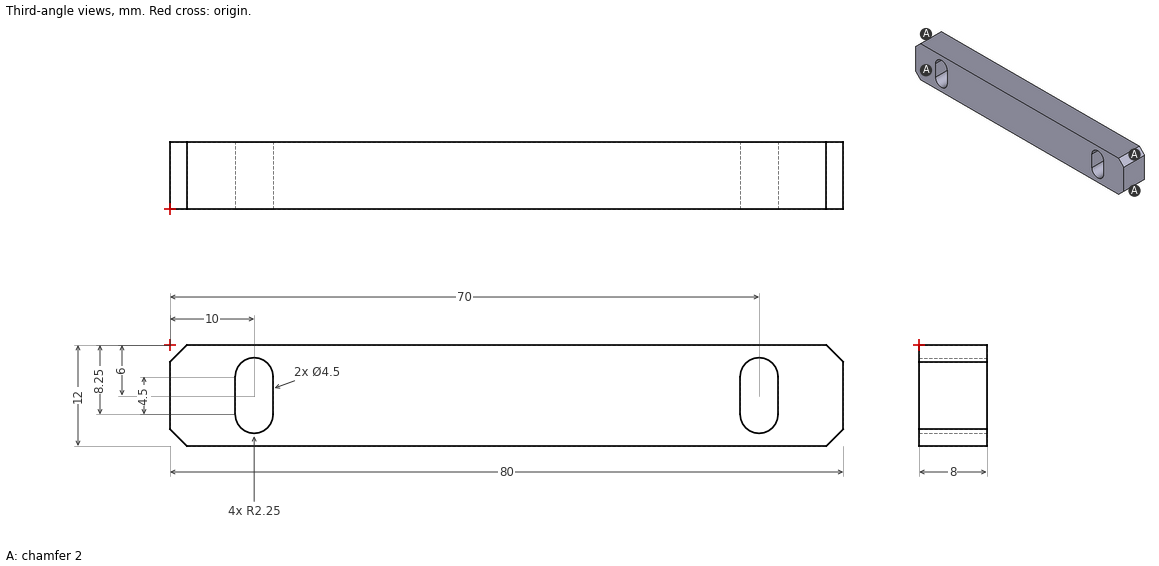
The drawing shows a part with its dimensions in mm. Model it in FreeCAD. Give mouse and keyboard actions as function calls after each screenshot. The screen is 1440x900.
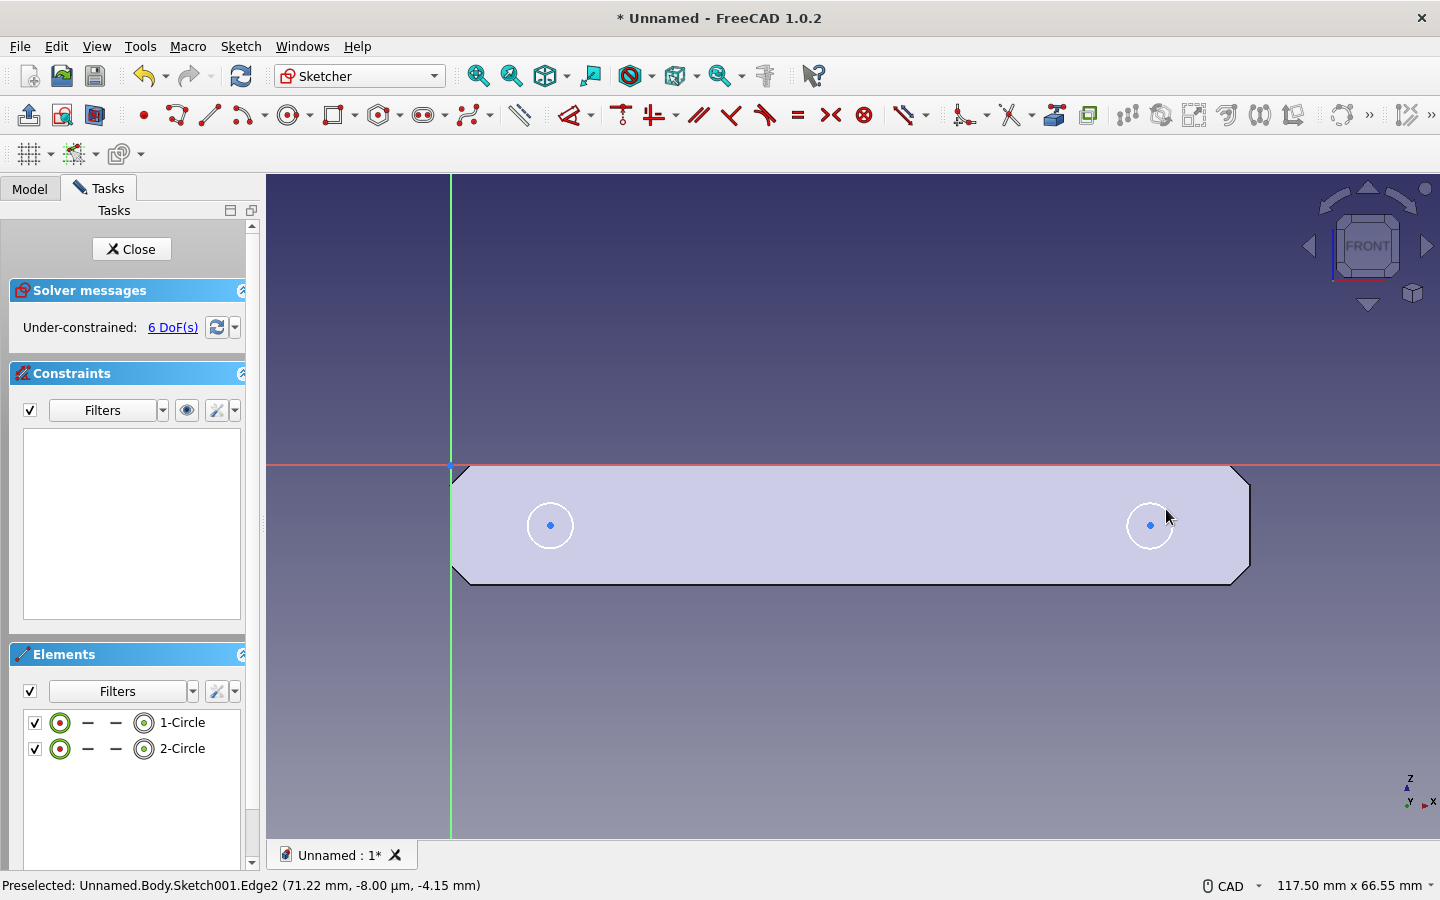
click(566, 510)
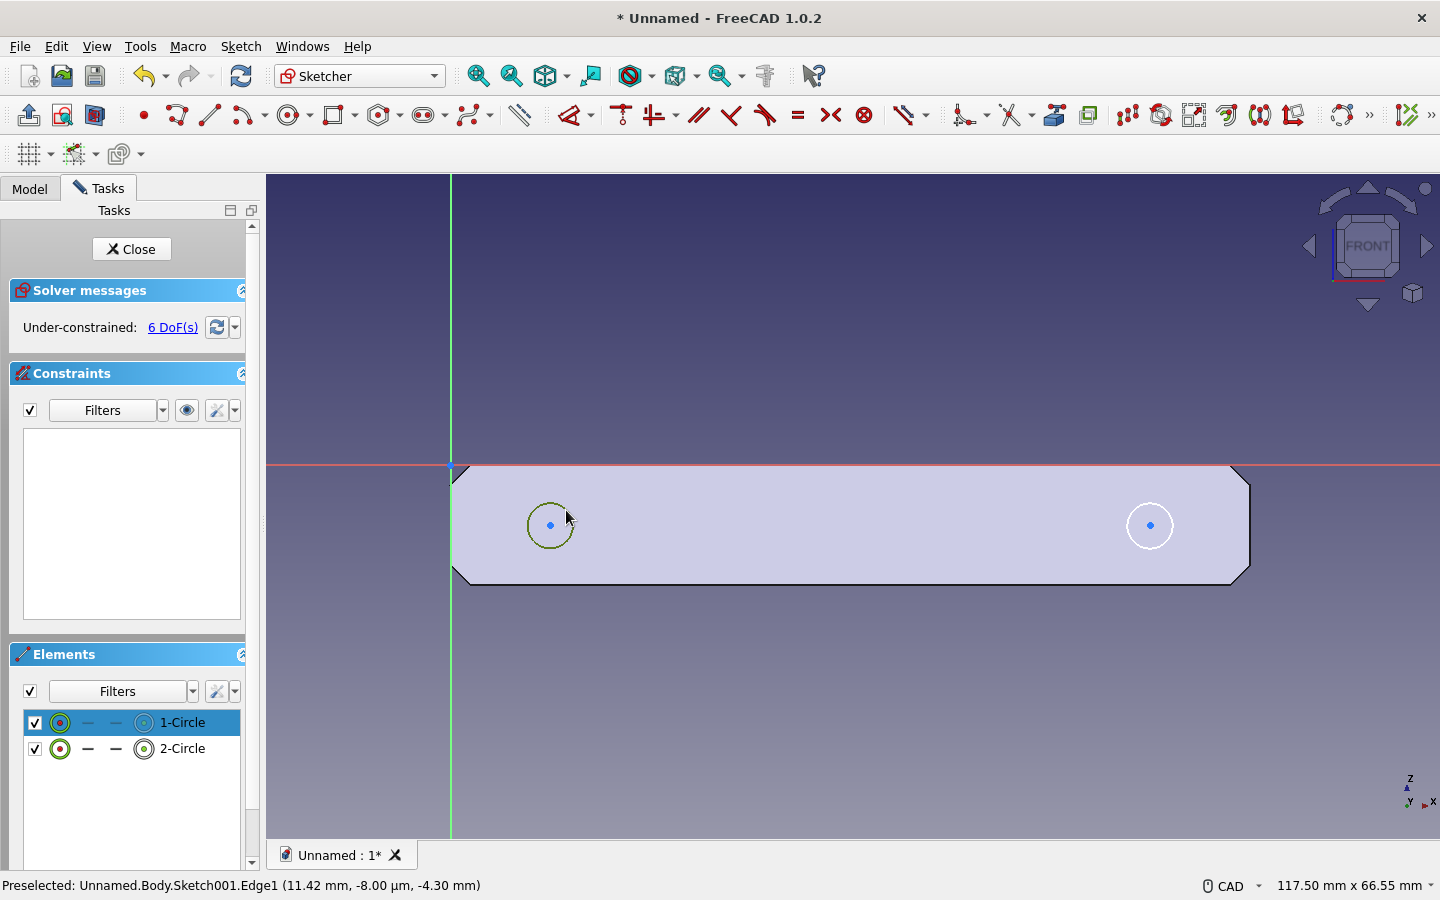
click(1166, 510)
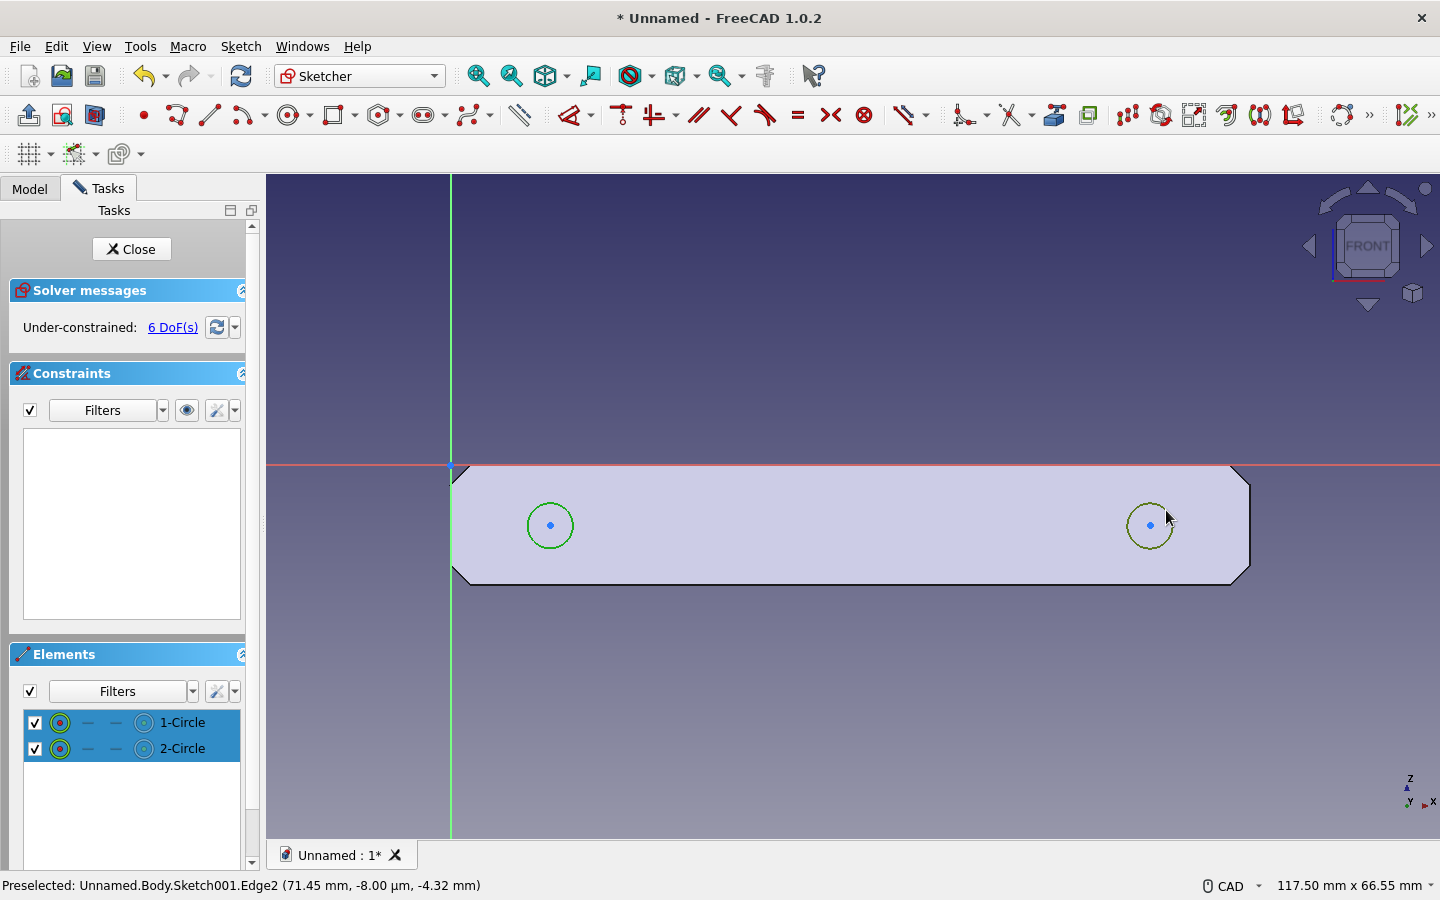
key(e)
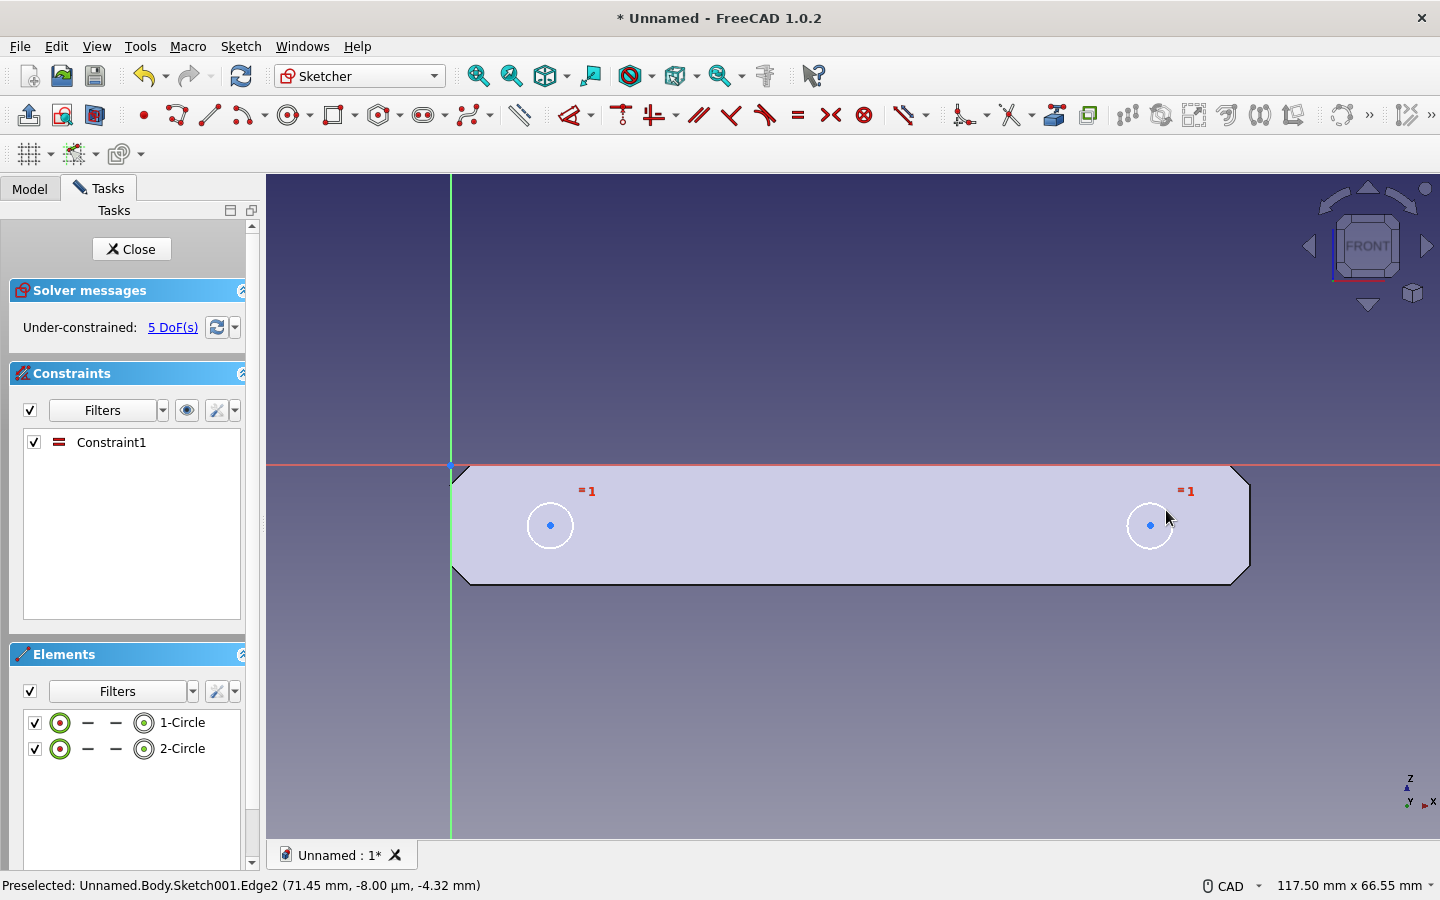
click(550, 526)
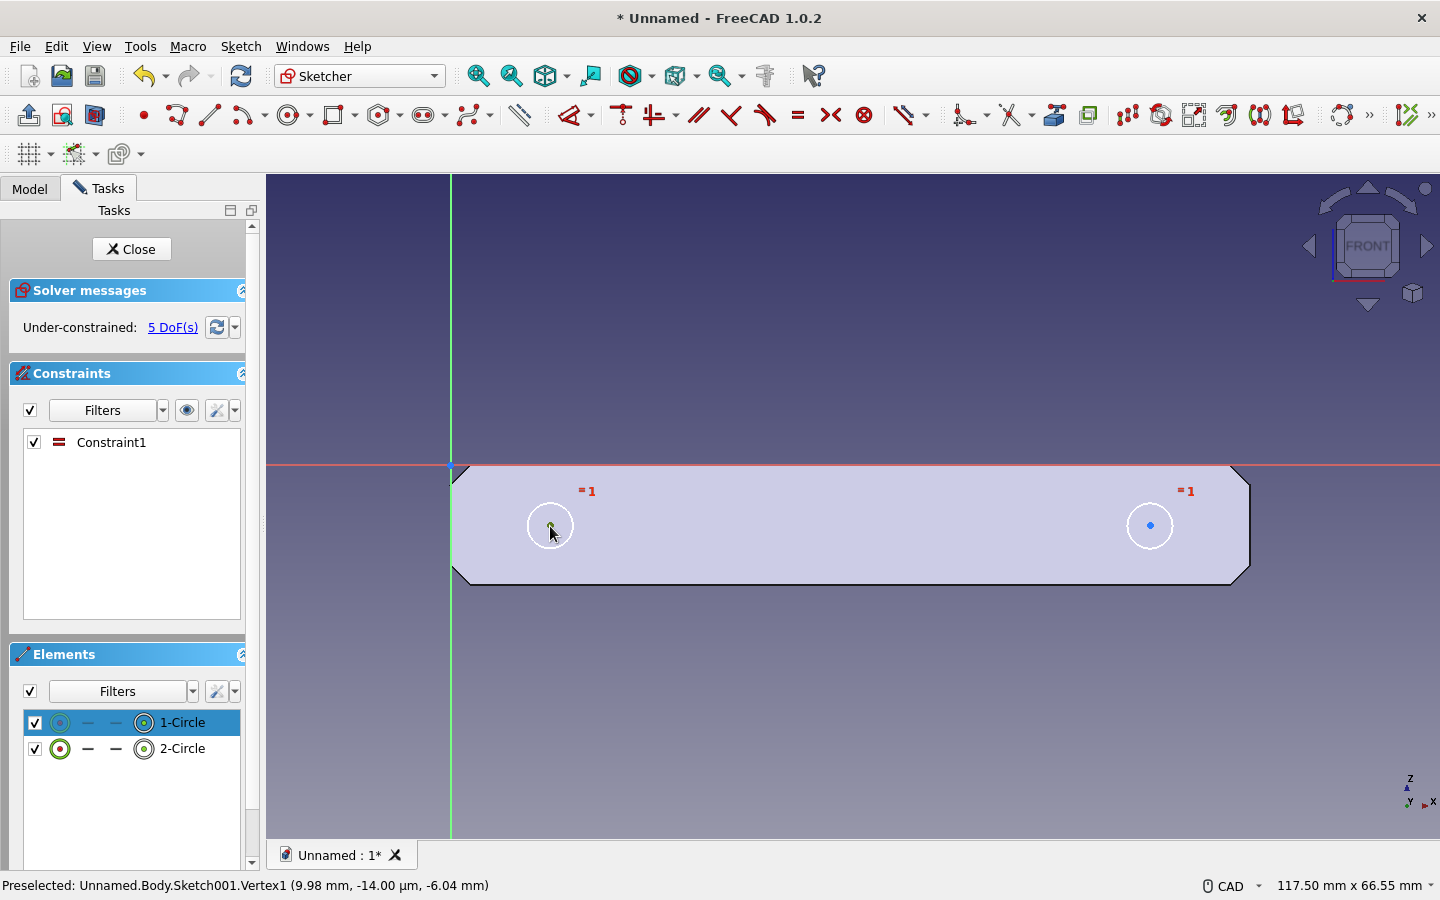
click(1150, 526)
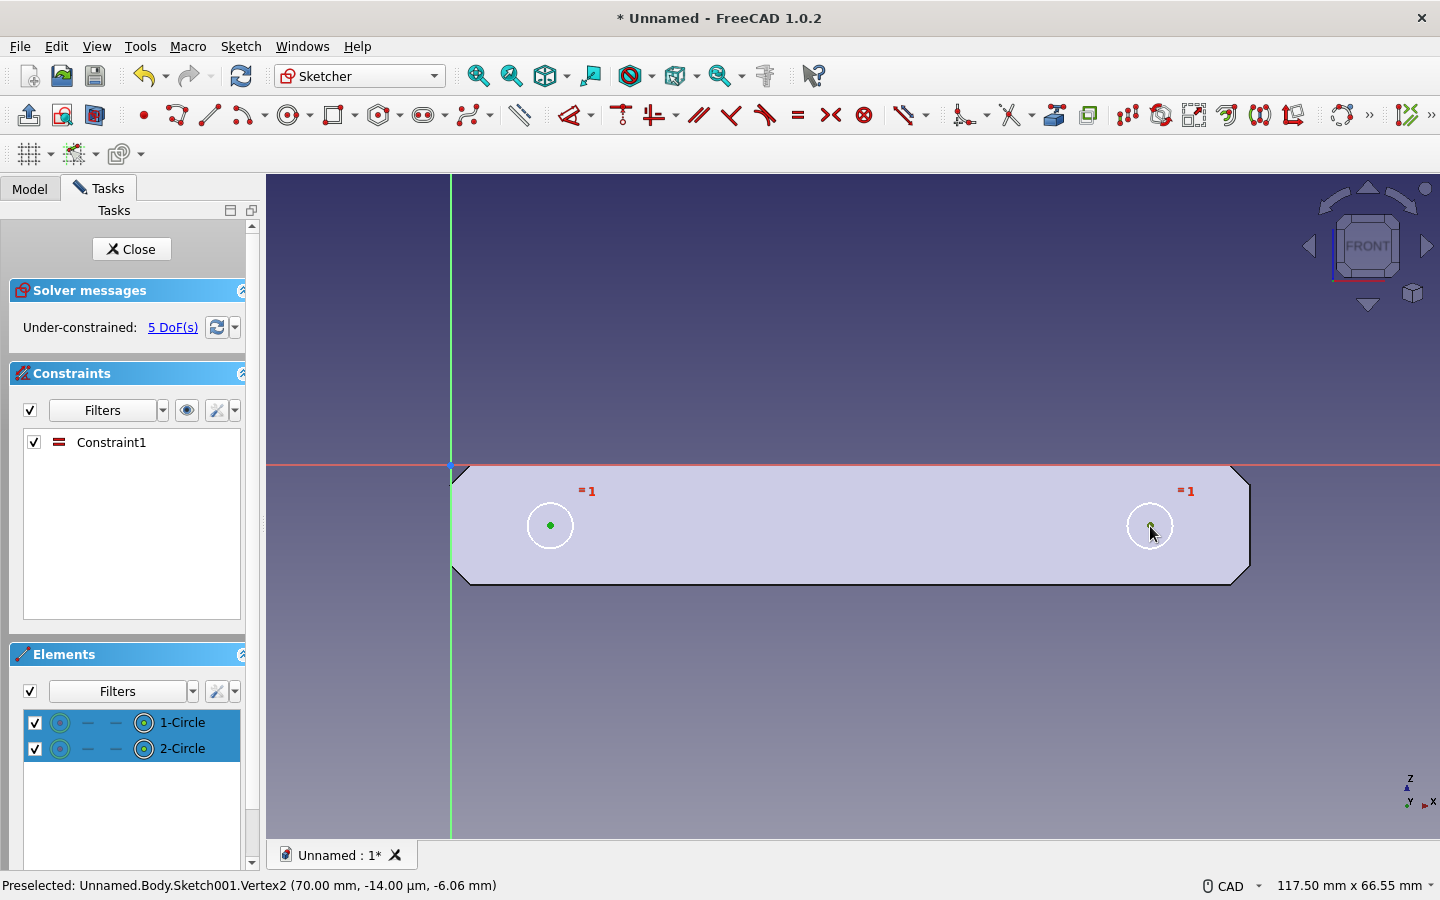
key(h)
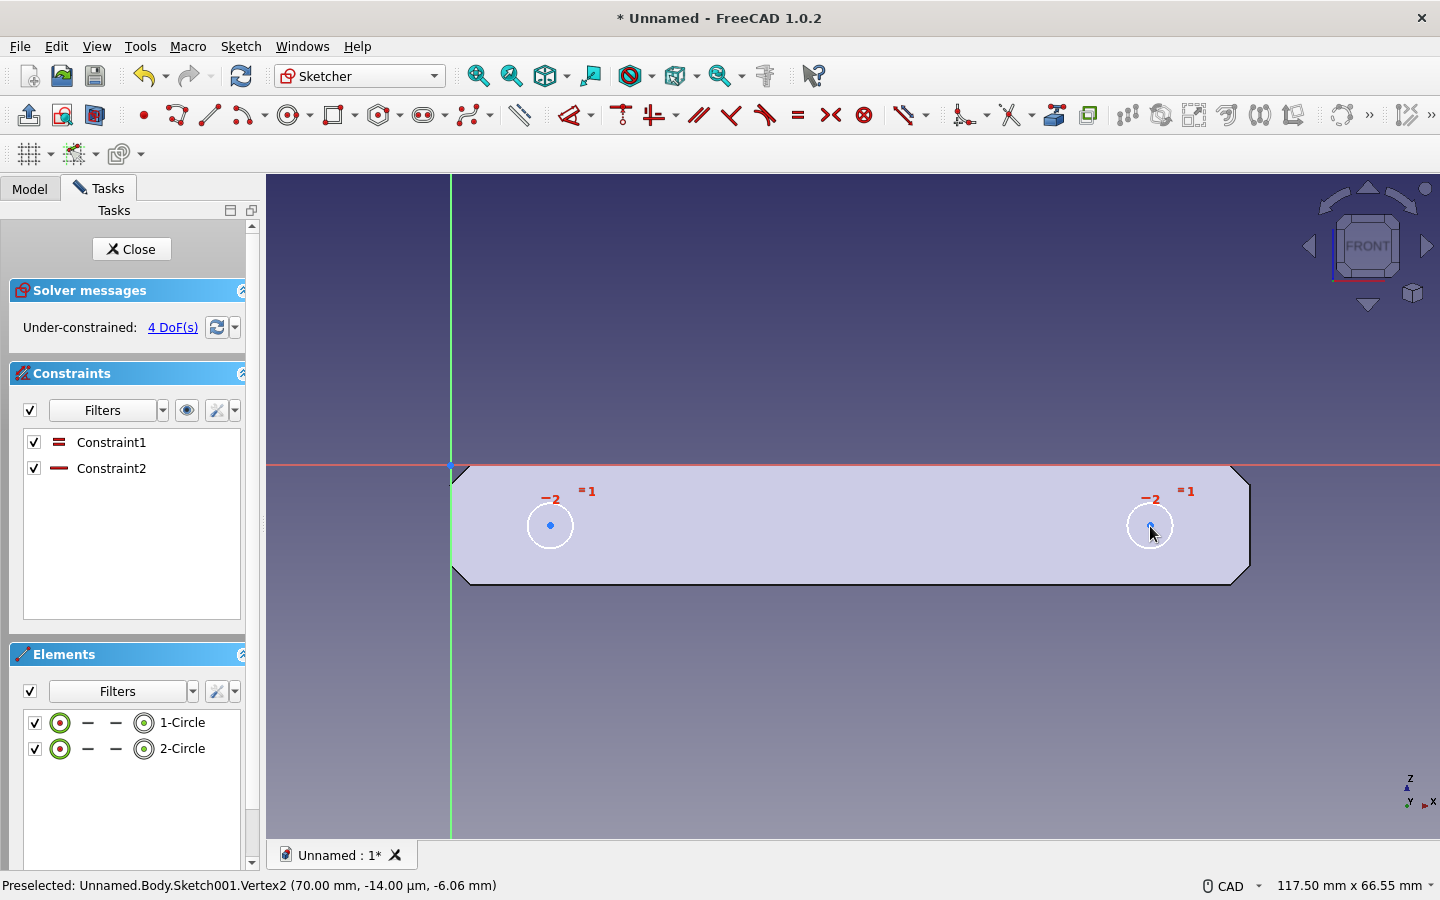
key(d)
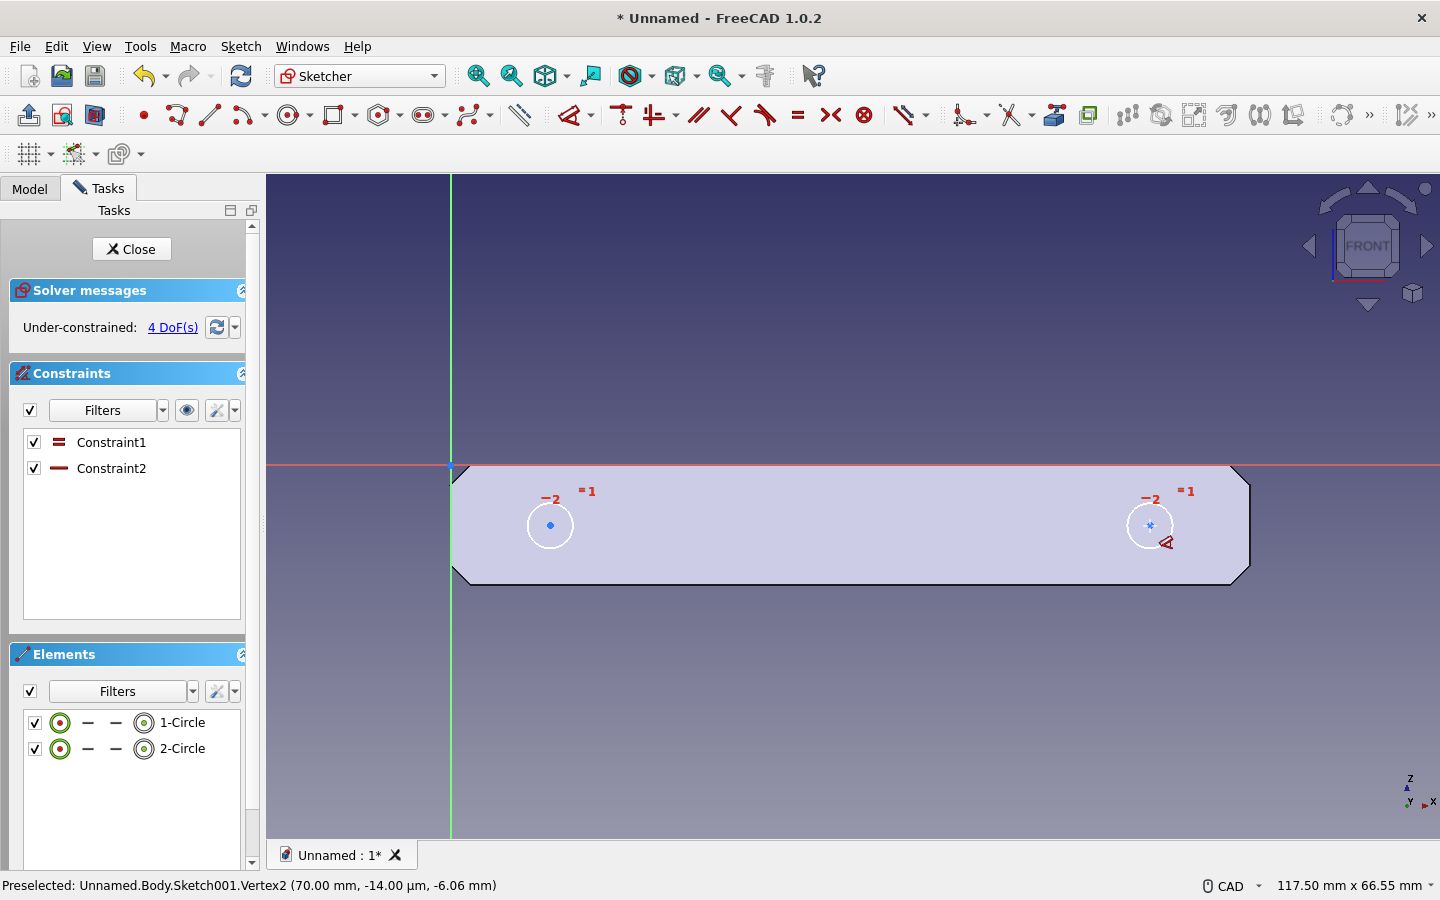
click(566, 510)
click(589, 487)